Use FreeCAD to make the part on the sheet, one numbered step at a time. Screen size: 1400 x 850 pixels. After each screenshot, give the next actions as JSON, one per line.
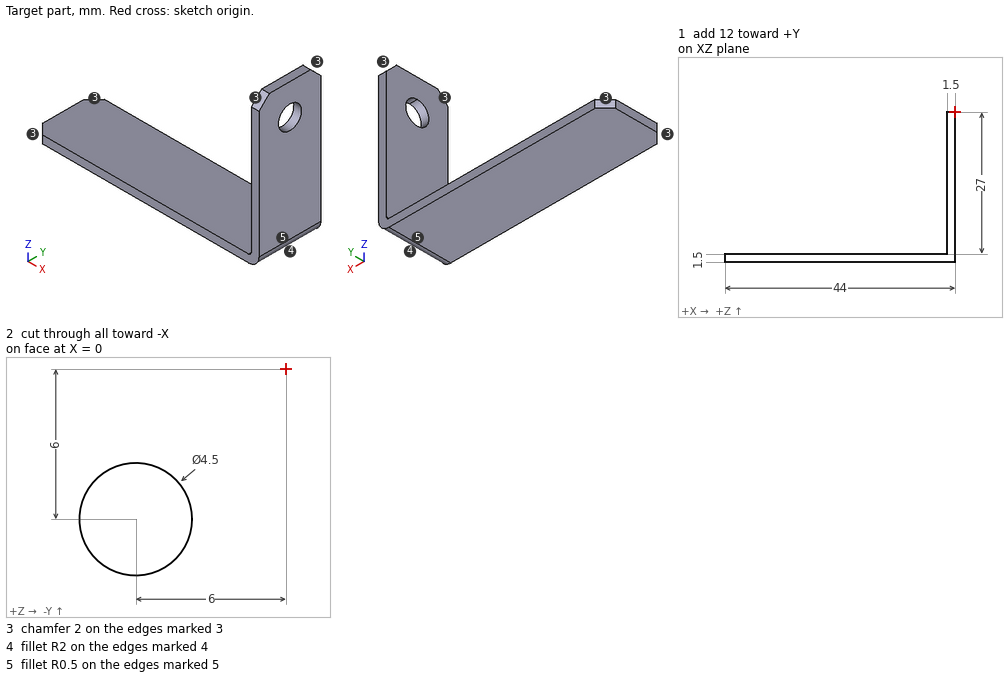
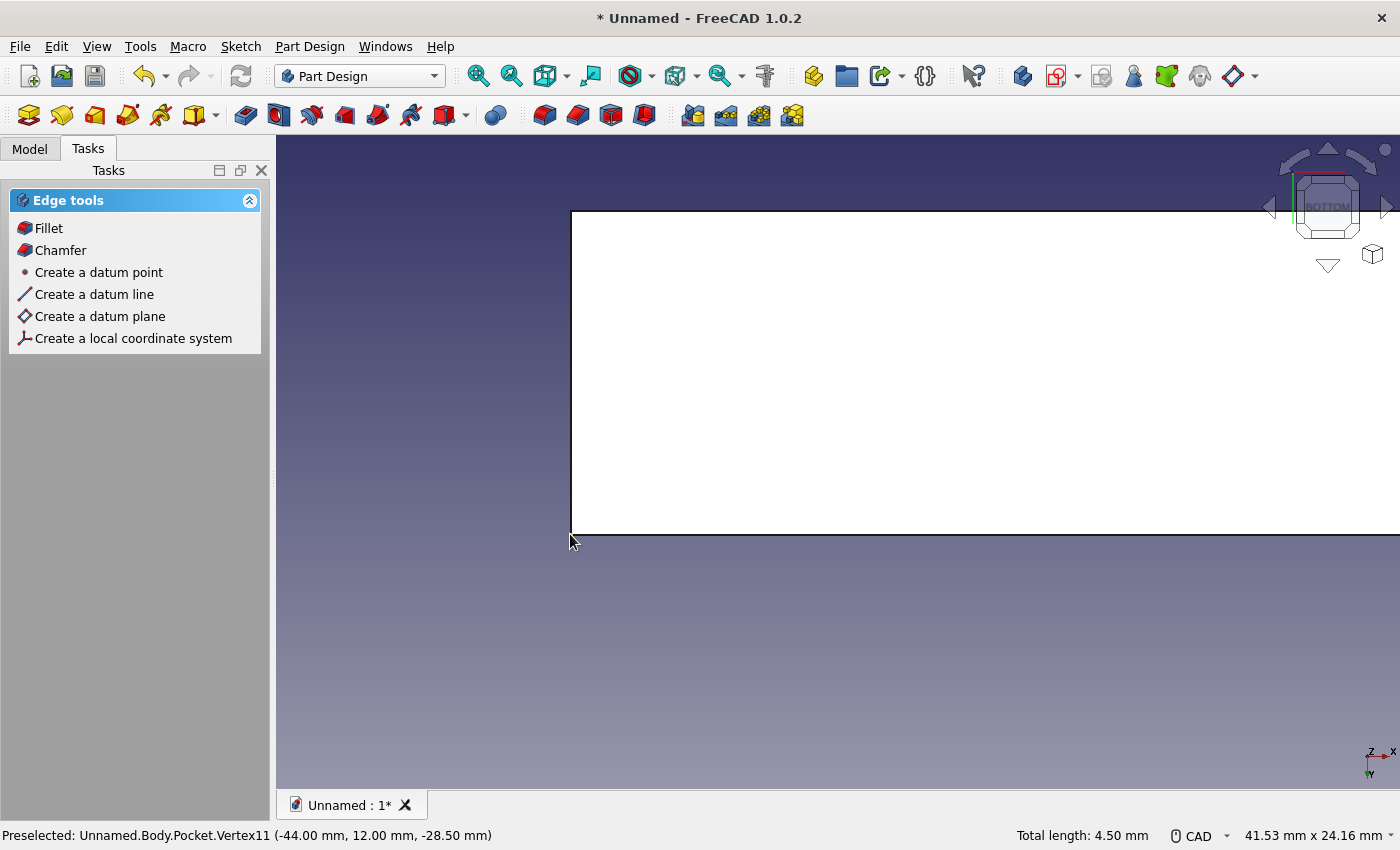
{"action": "left_click", "coordinate": [479, 76]}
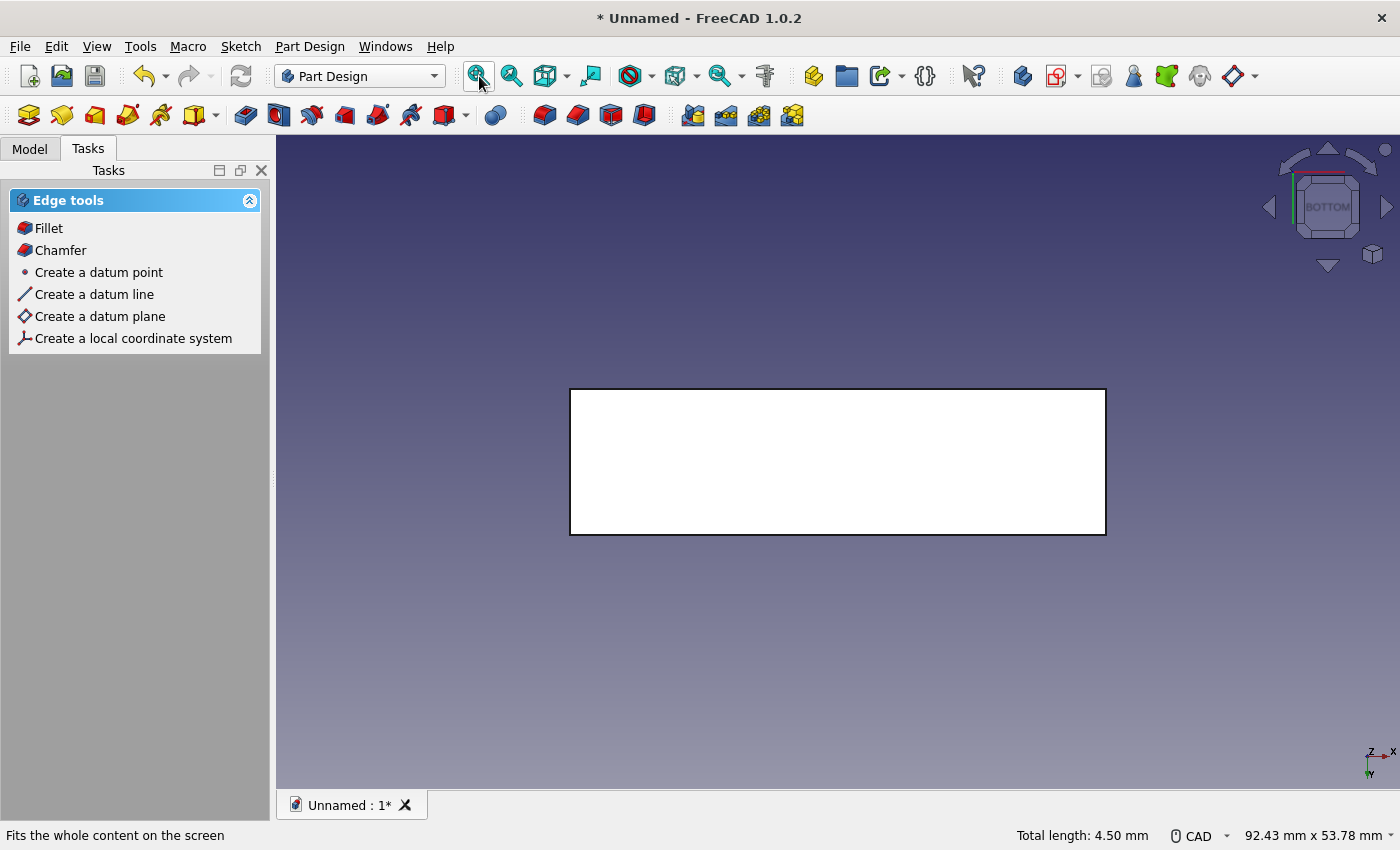
{"action": "key", "text": "4"}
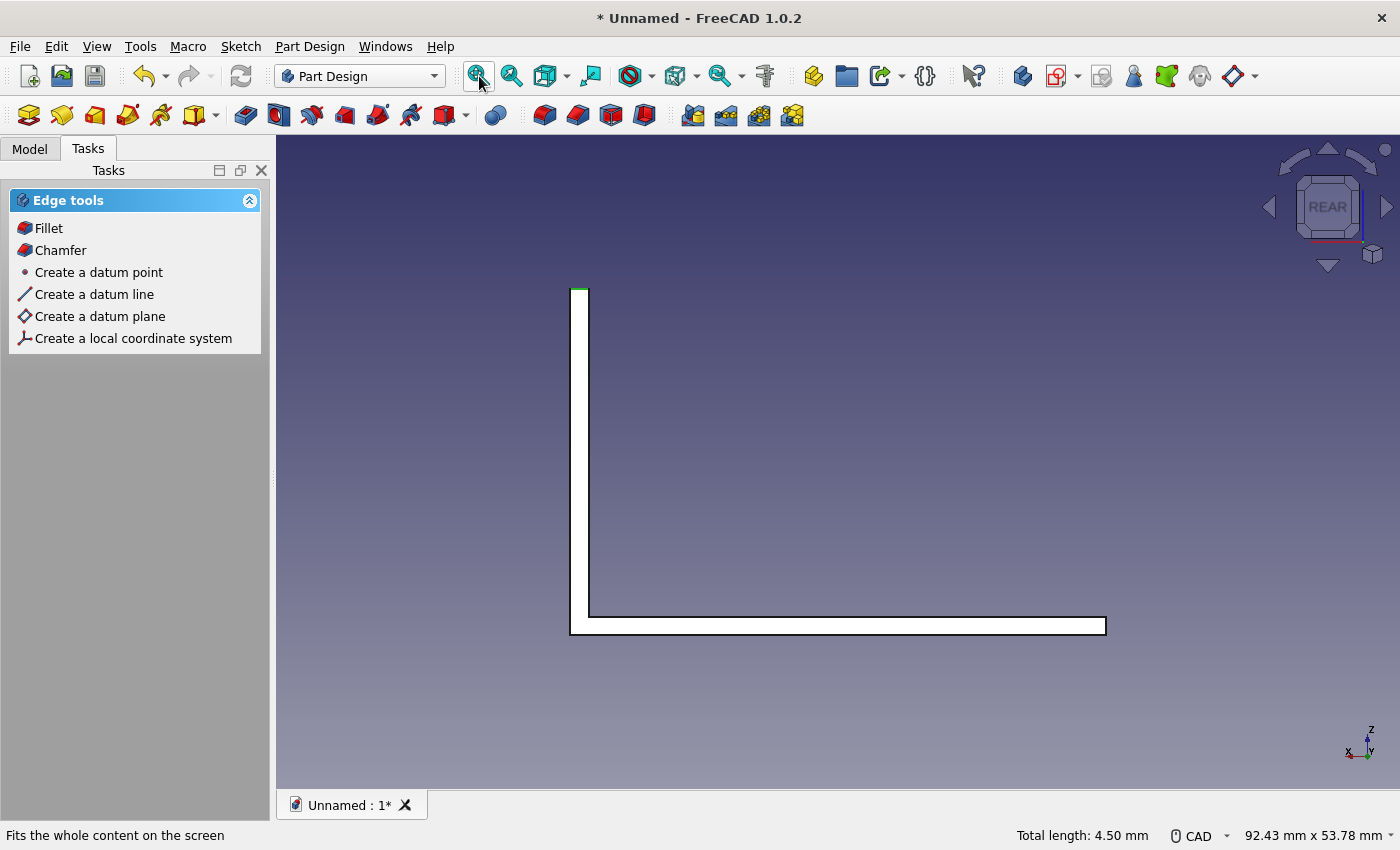
{"action": "left_click", "coordinate": [1106, 625], "text": "ctrl"}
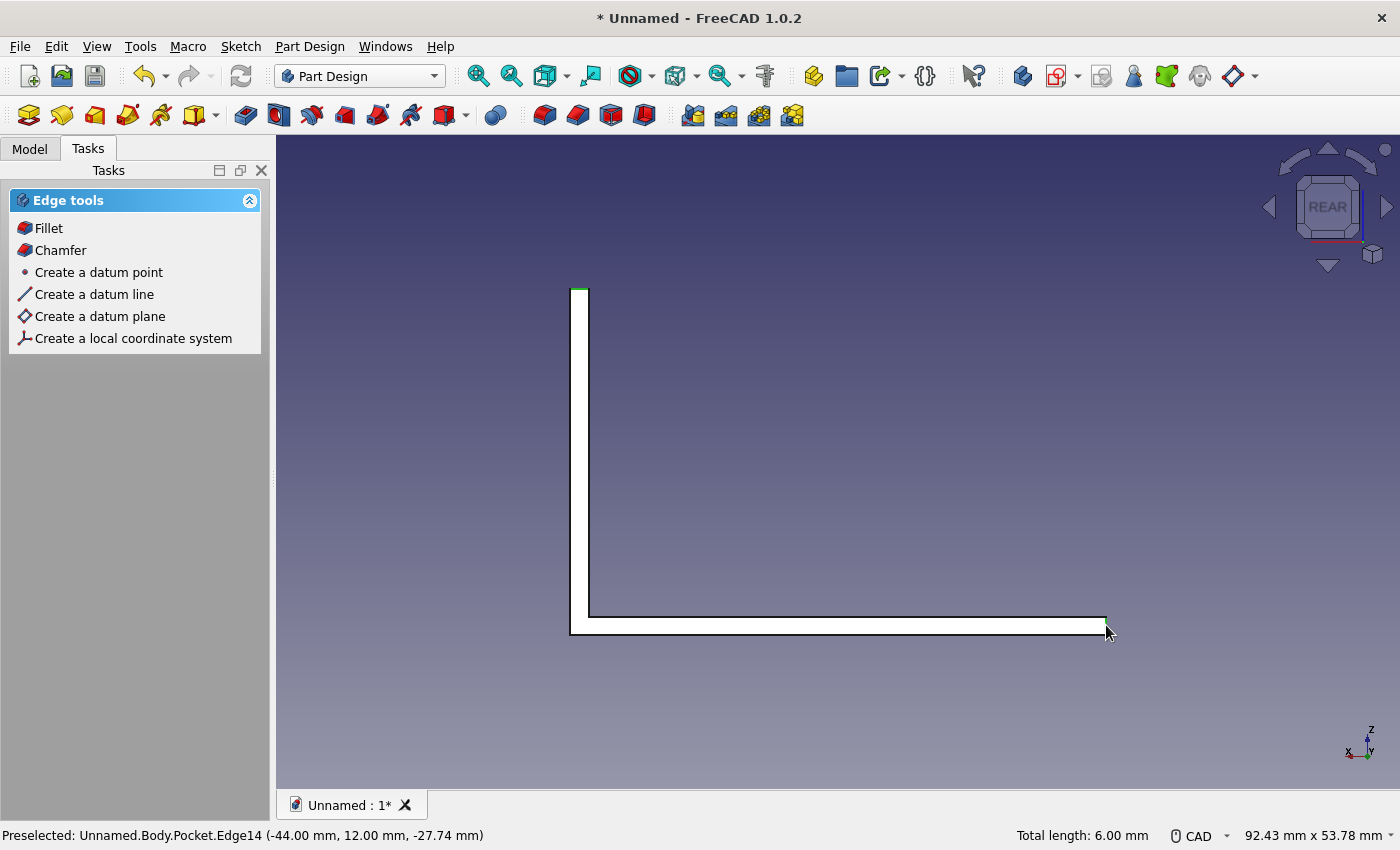
{"action": "left_click", "coordinate": [578, 116]}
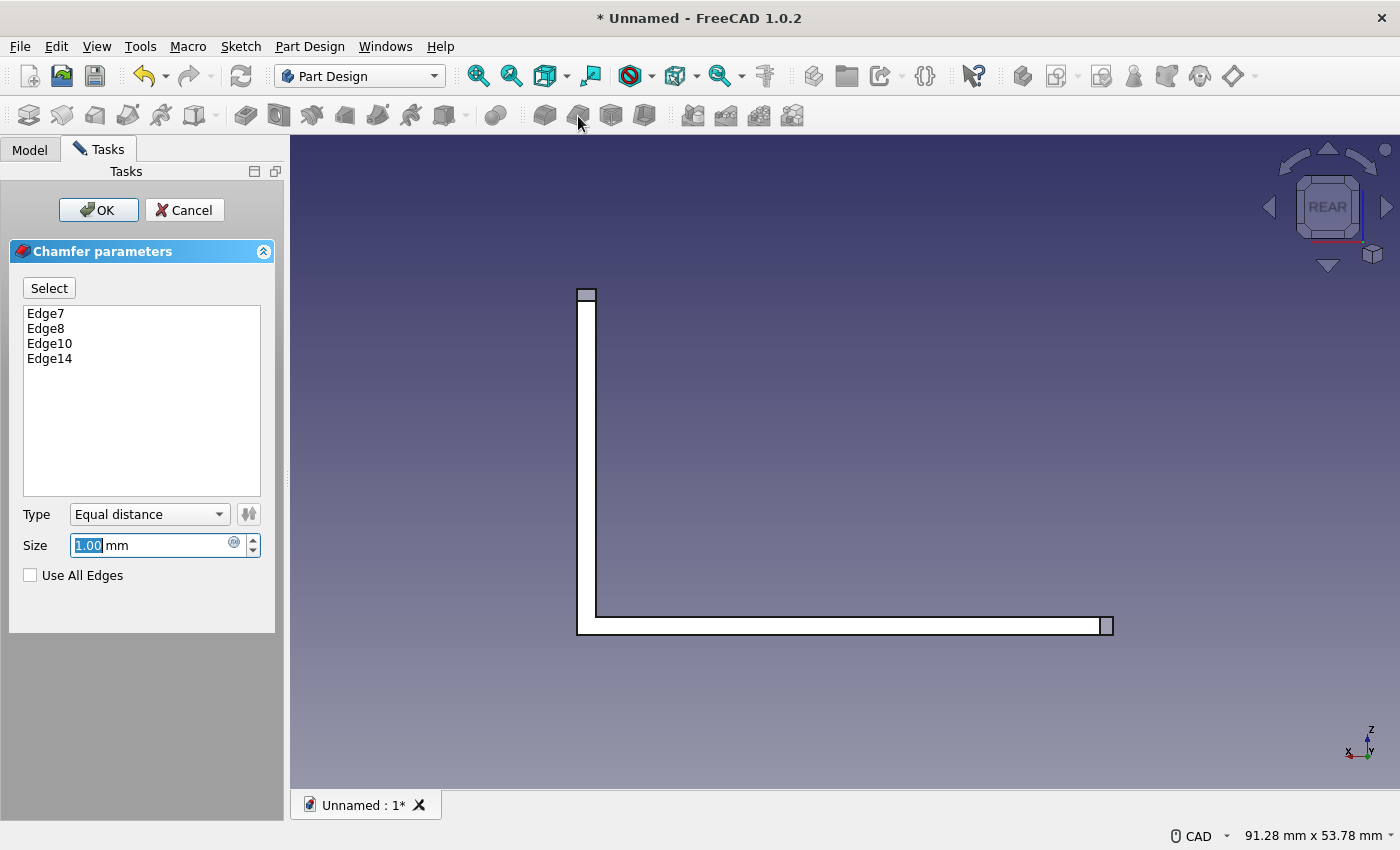
{"action": "type", "text": "2"}
{"action": "key", "text": "Tab"}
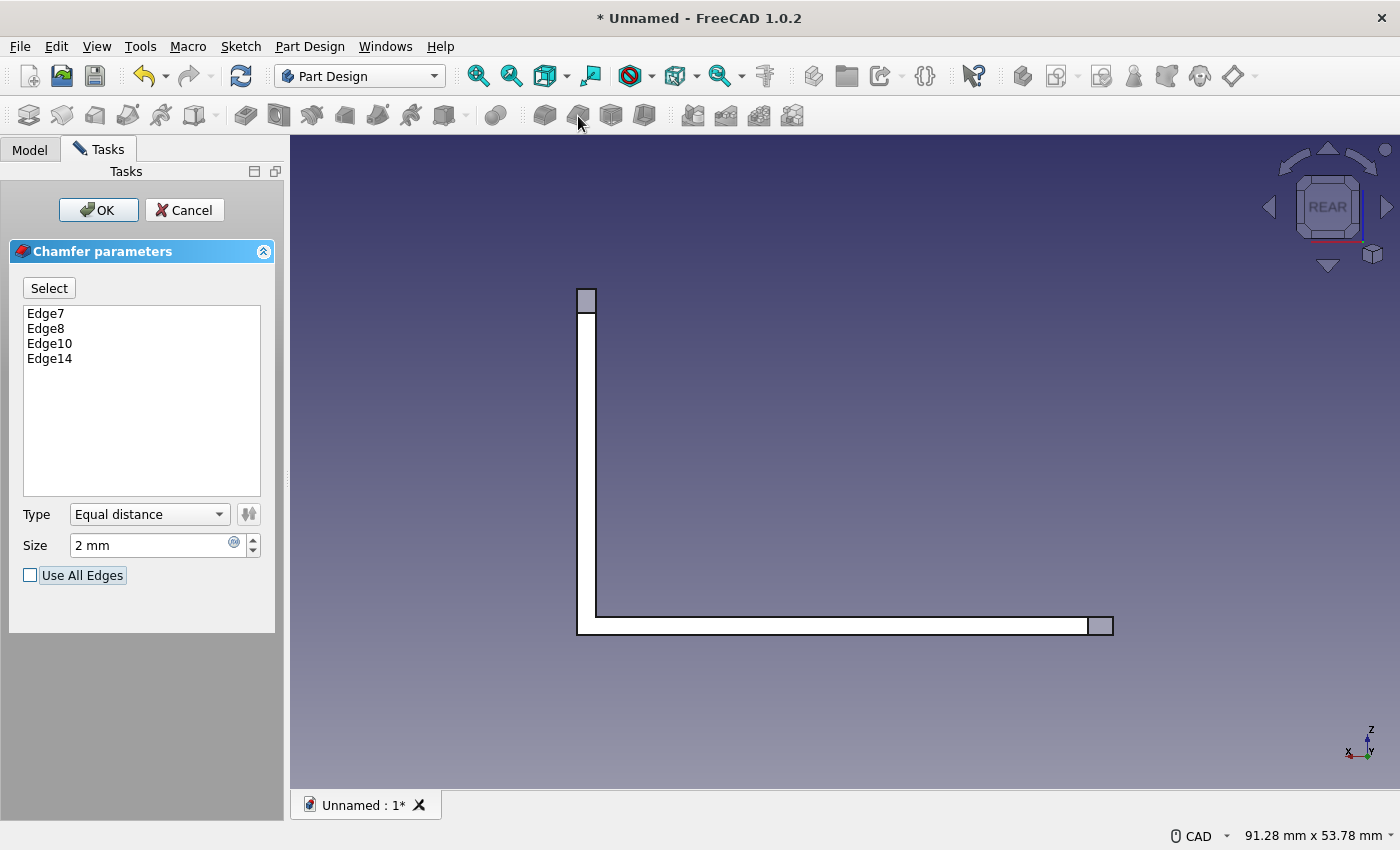
{"action": "left_click", "coordinate": [99, 210]}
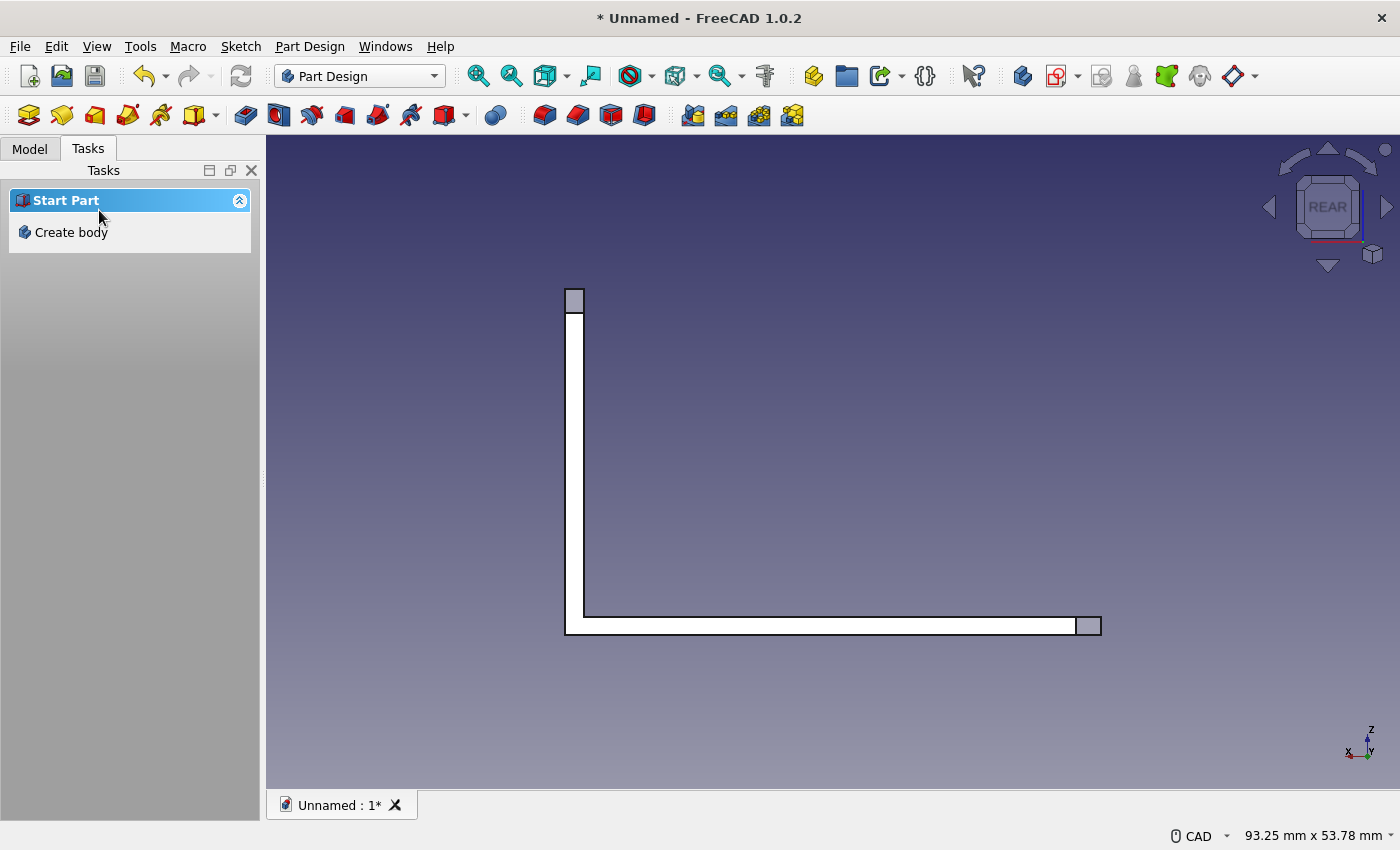
{"action": "key", "text": "0"}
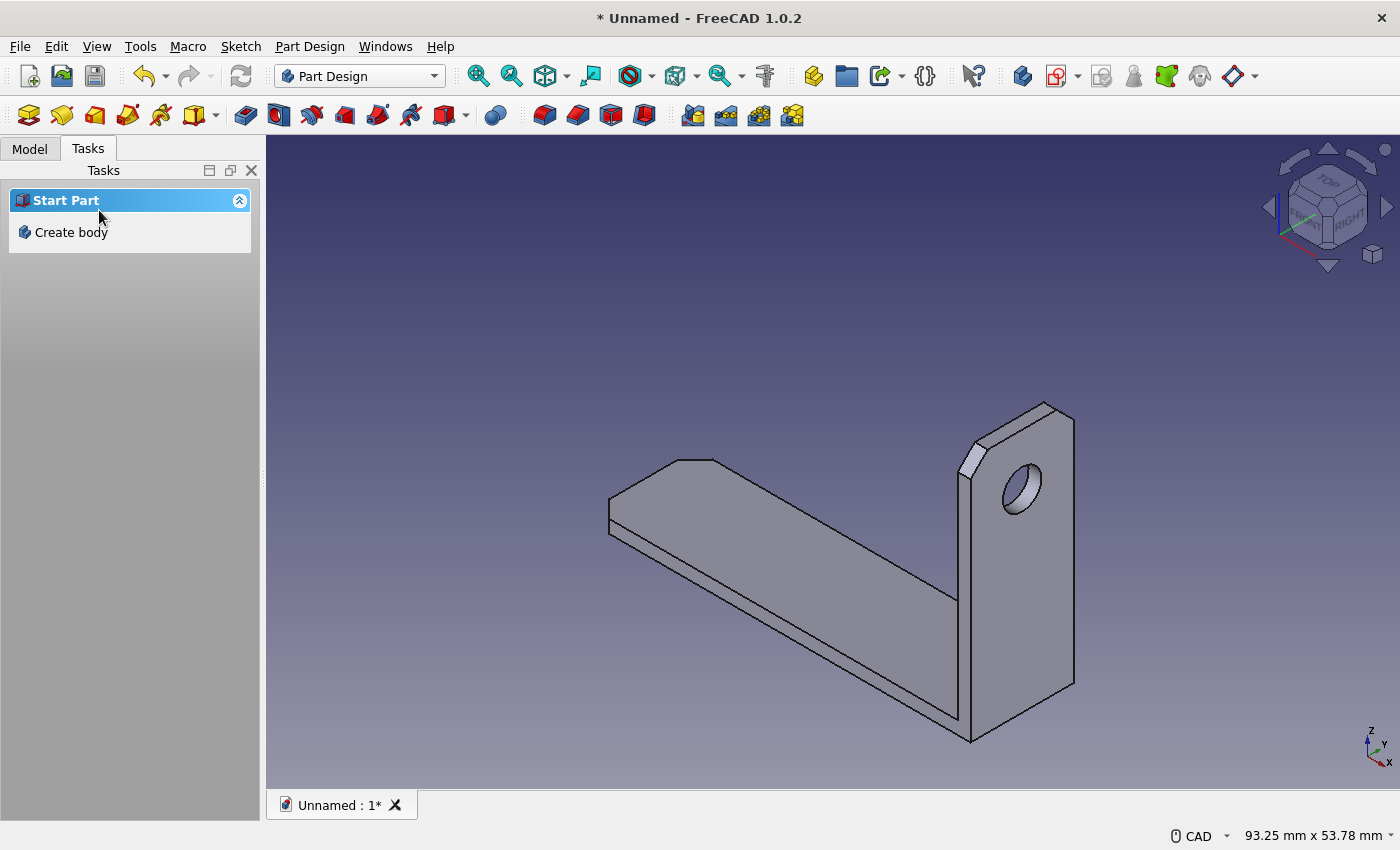
{"action": "key", "text": "2"}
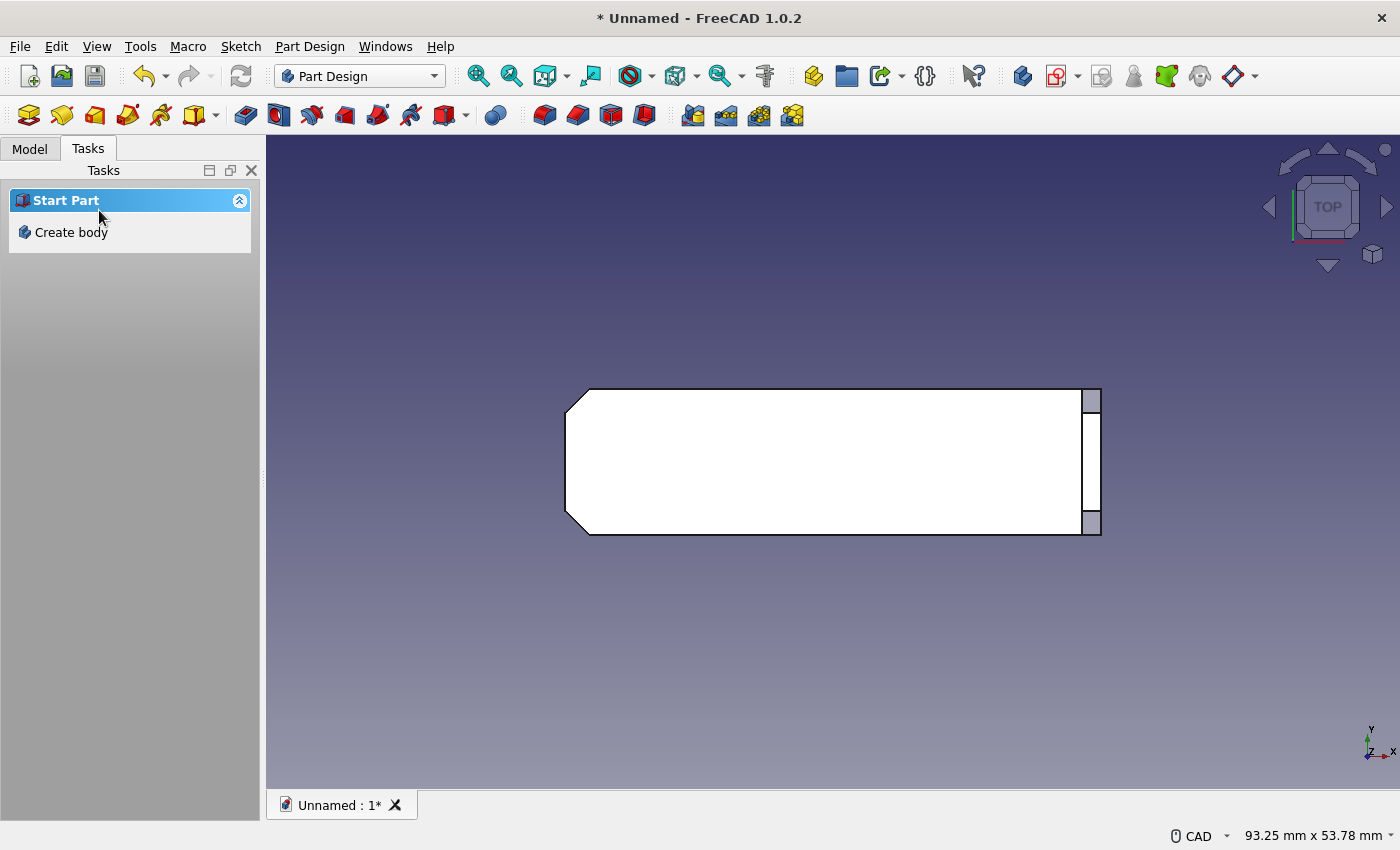
{"action": "key", "text": "1"}